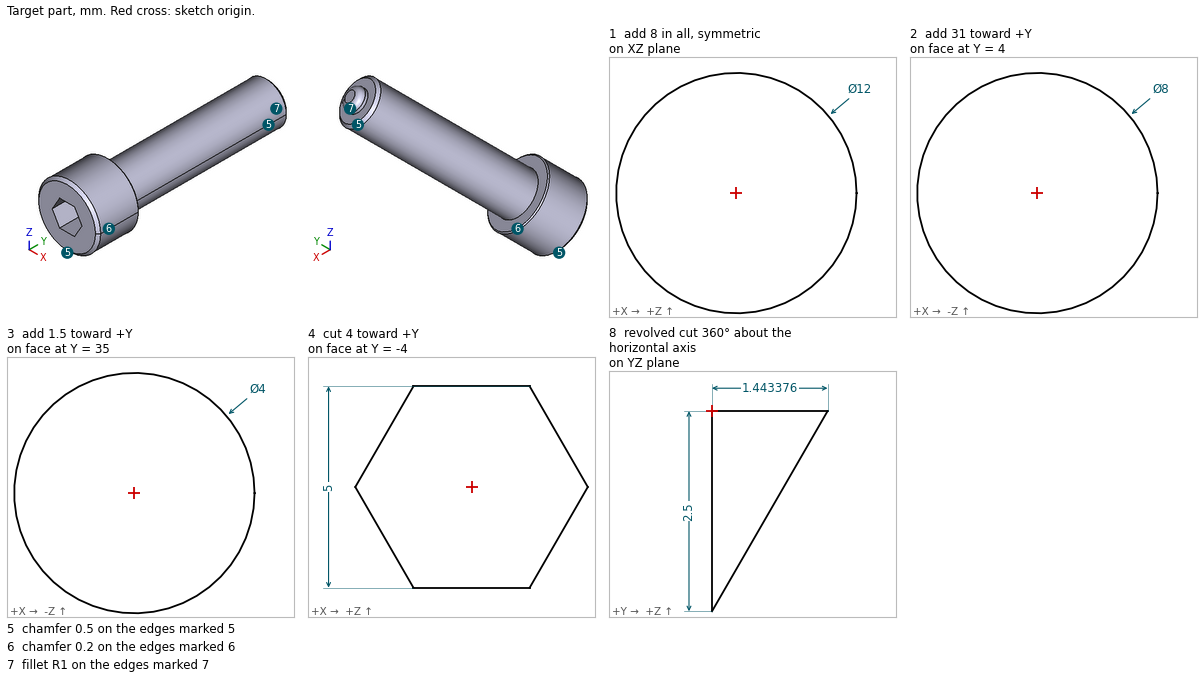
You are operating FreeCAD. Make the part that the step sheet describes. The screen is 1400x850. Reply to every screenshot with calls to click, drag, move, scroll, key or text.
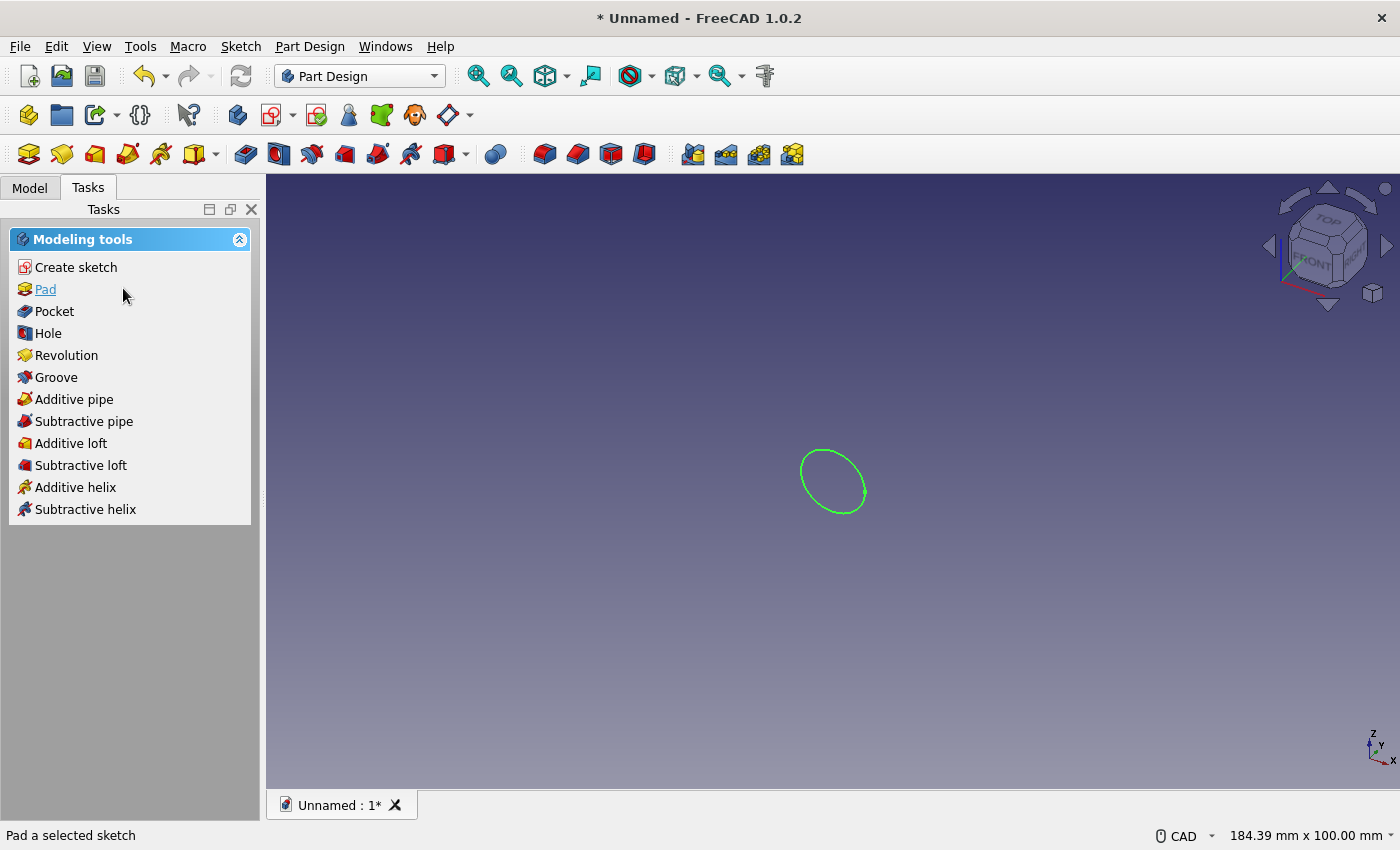
click(29, 154)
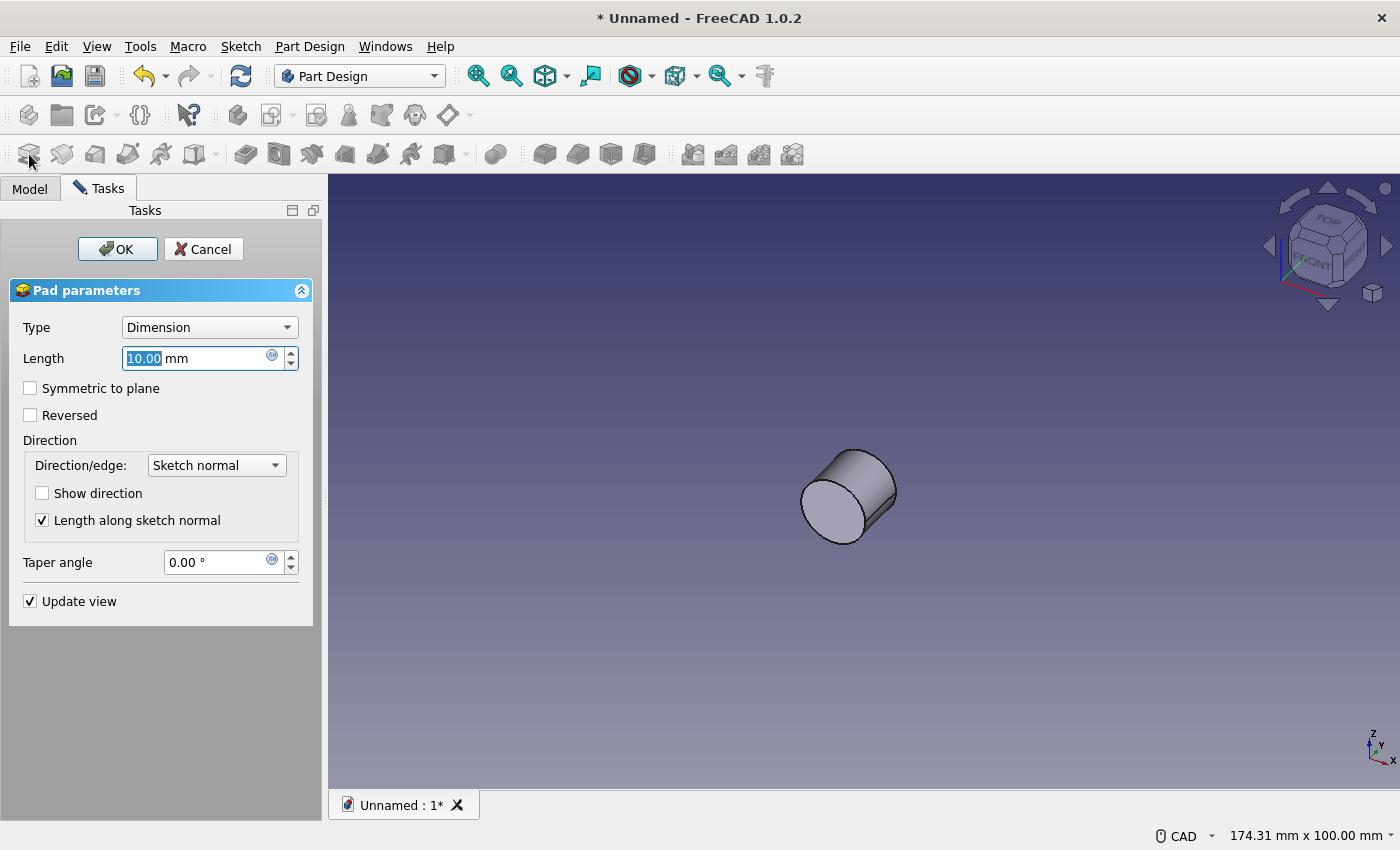
text(8)
key(Tab)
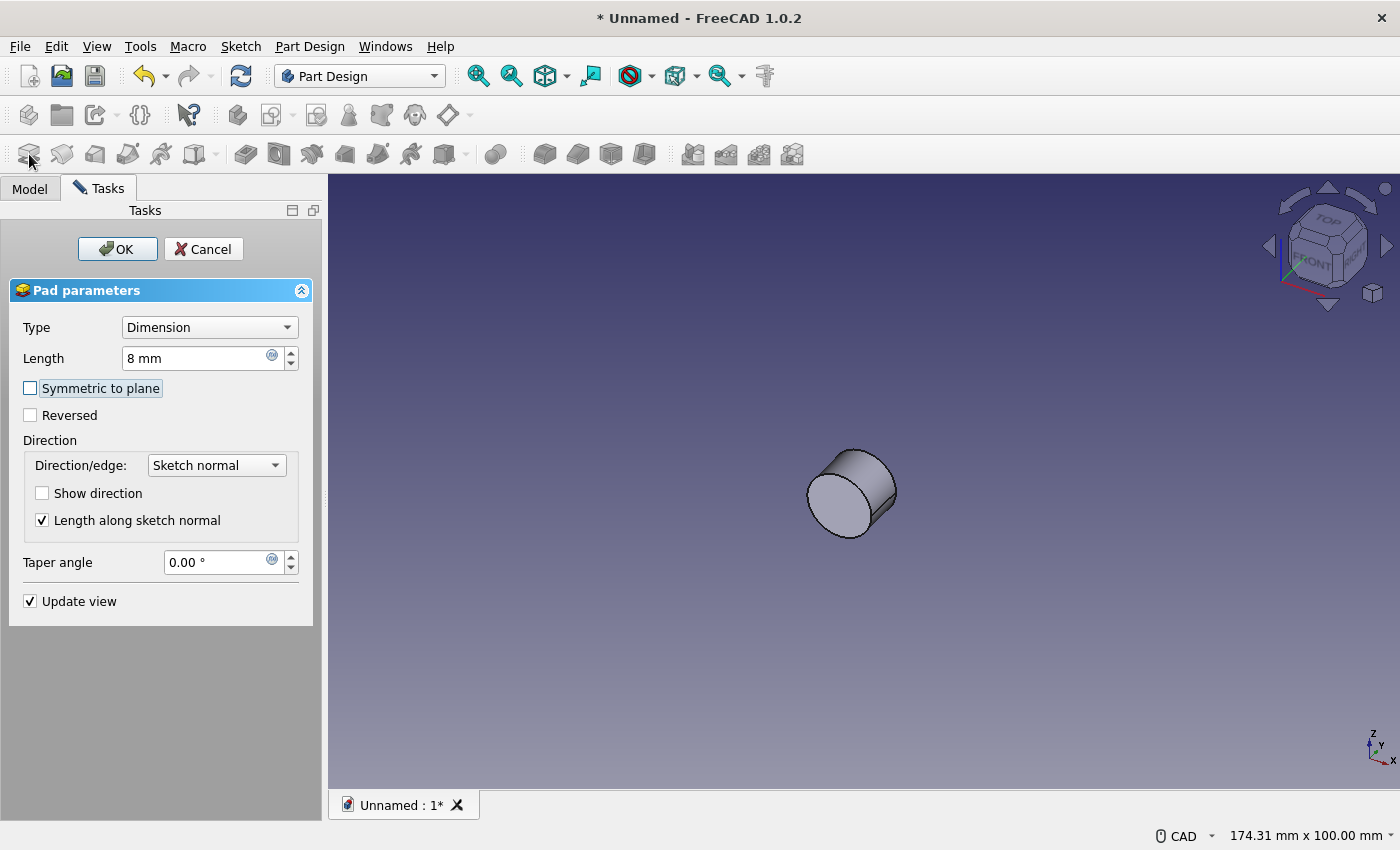
click(31, 388)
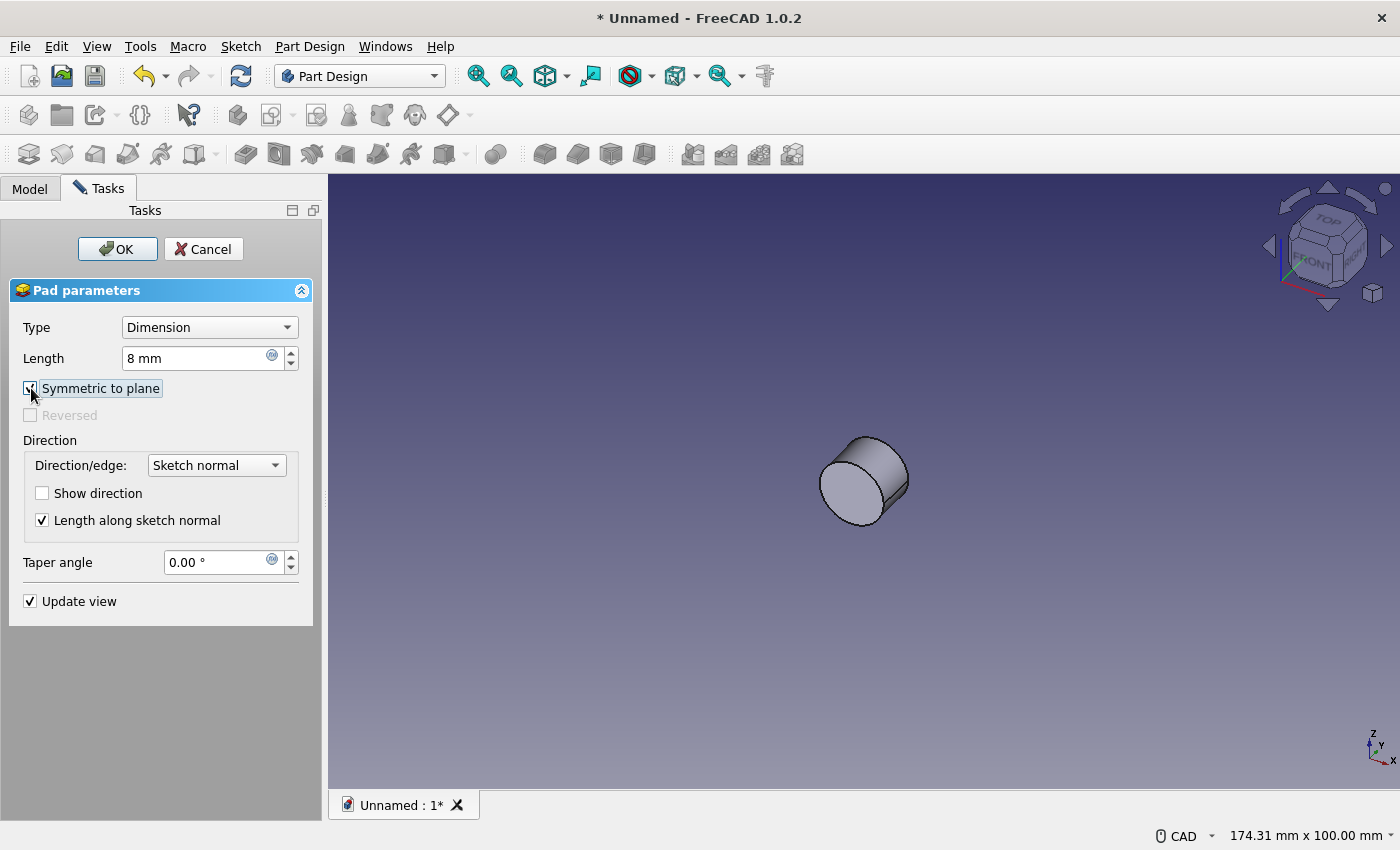
click(118, 249)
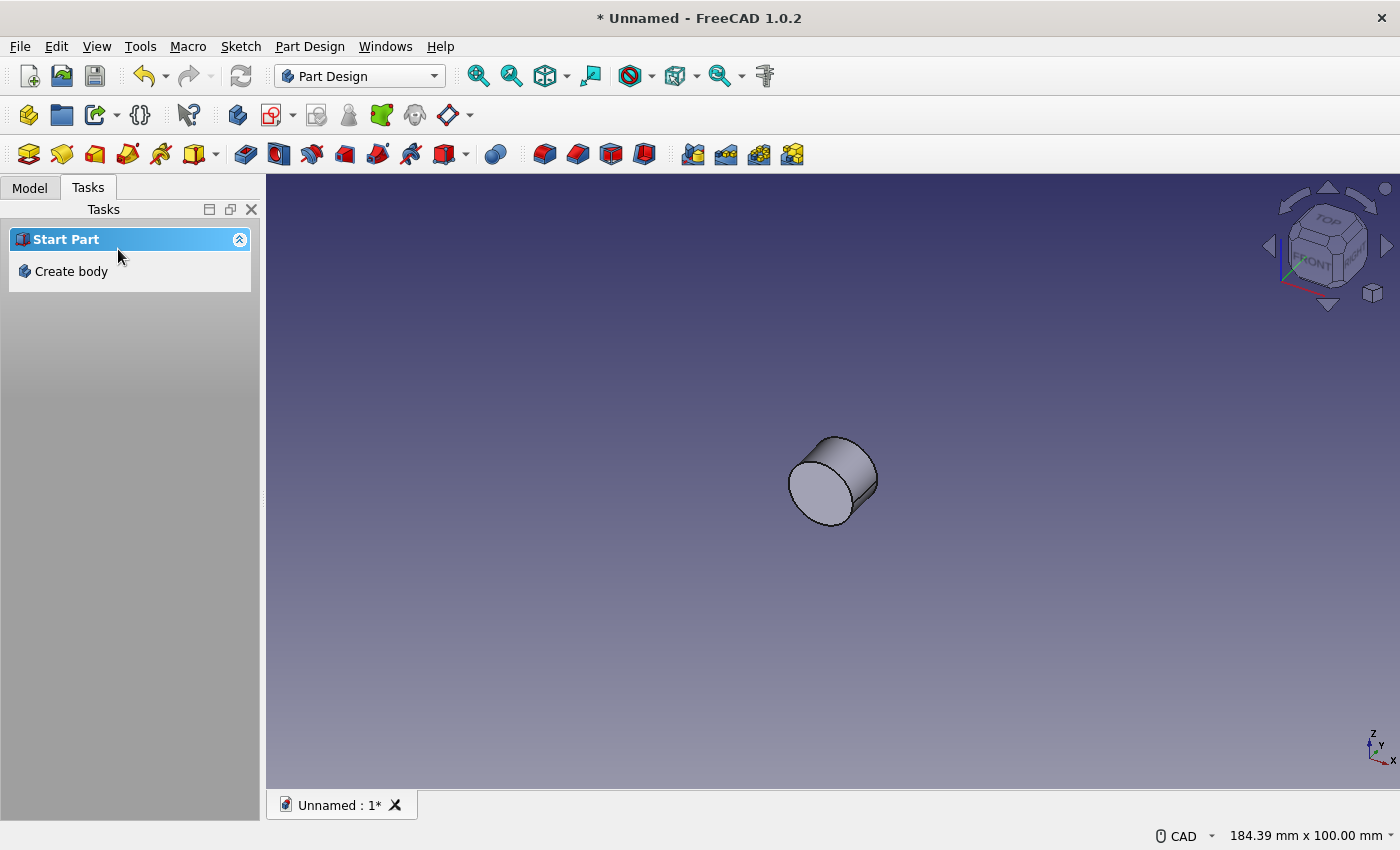
key(v)
key(f)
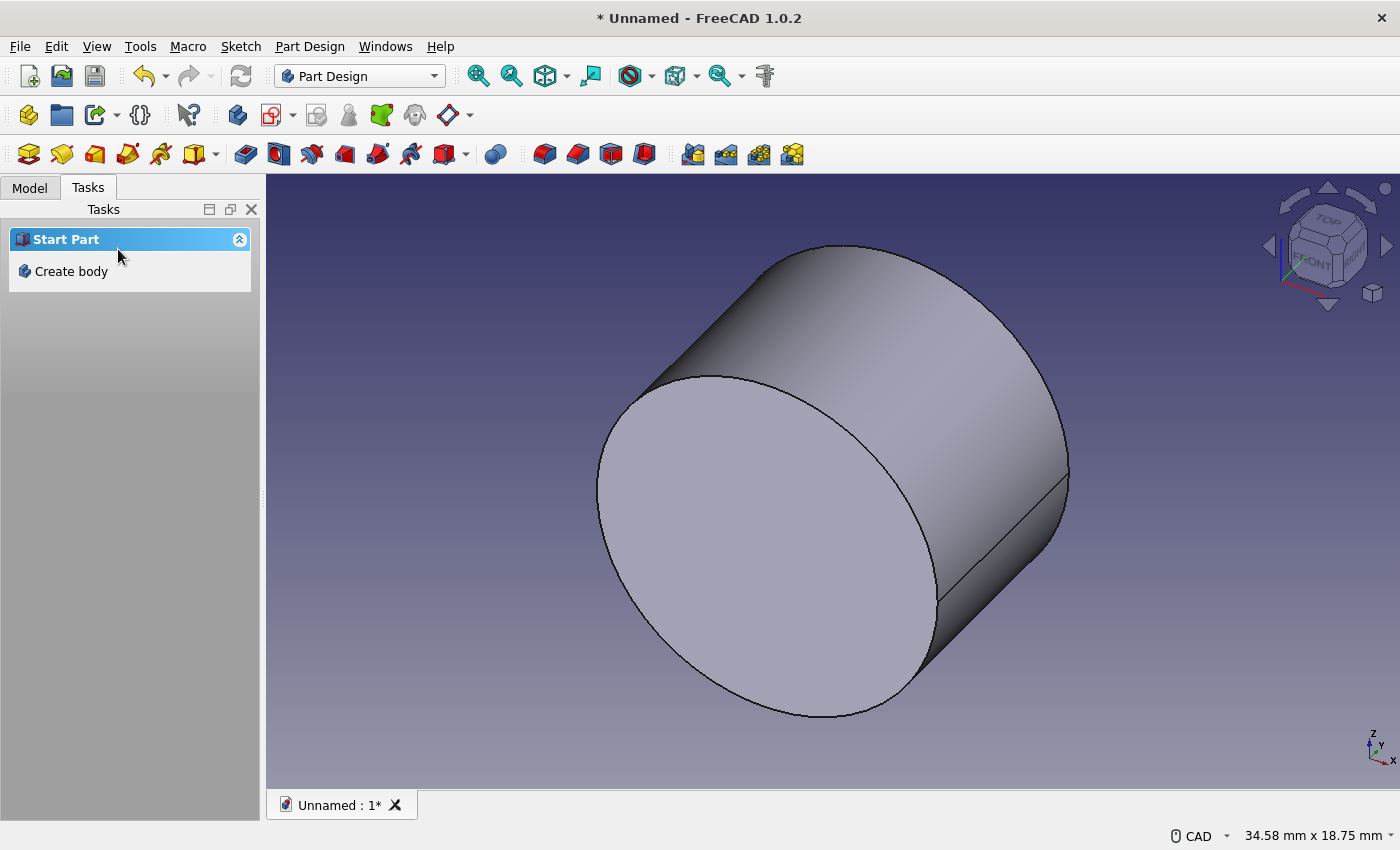
key(4)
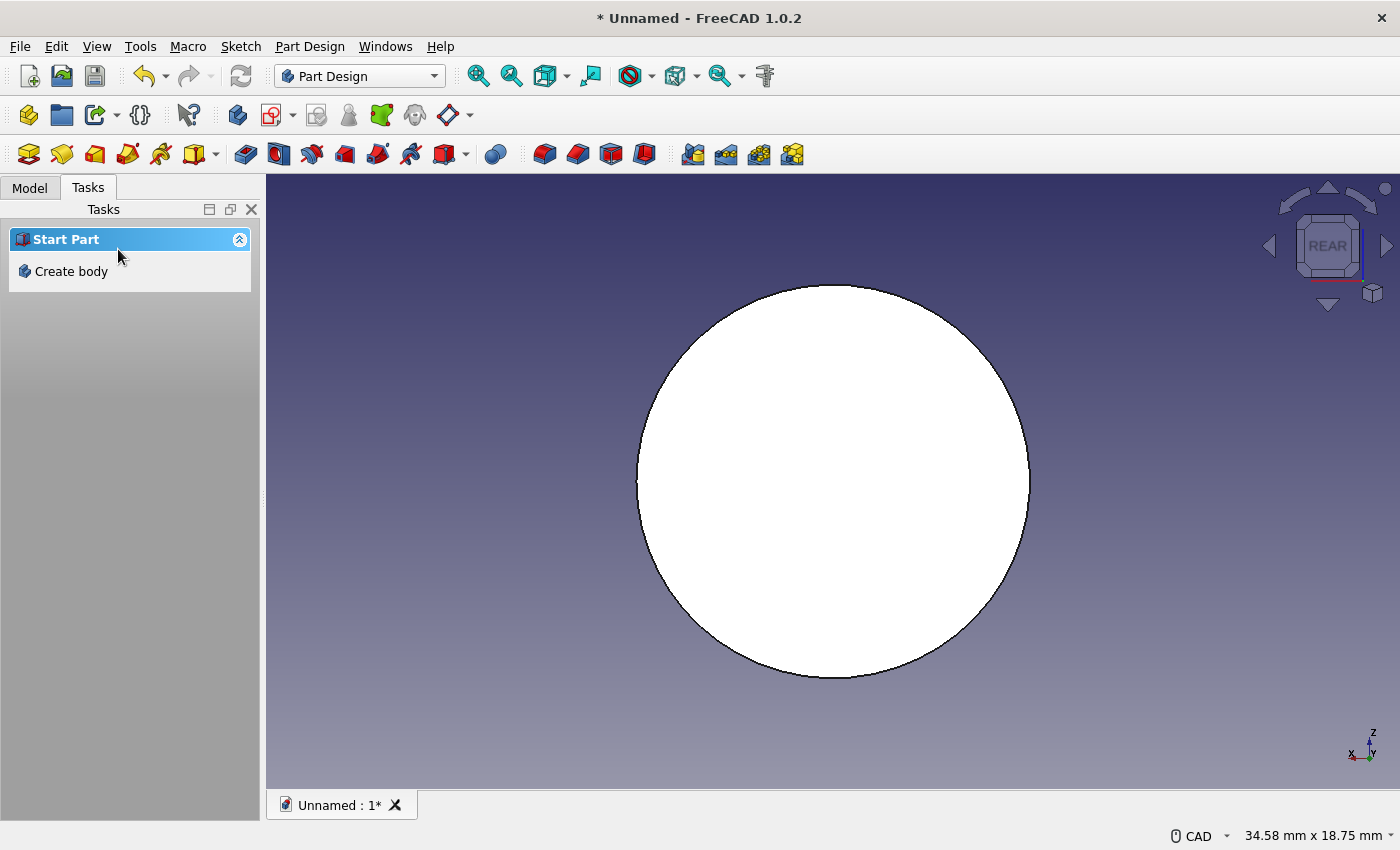
click(833, 481)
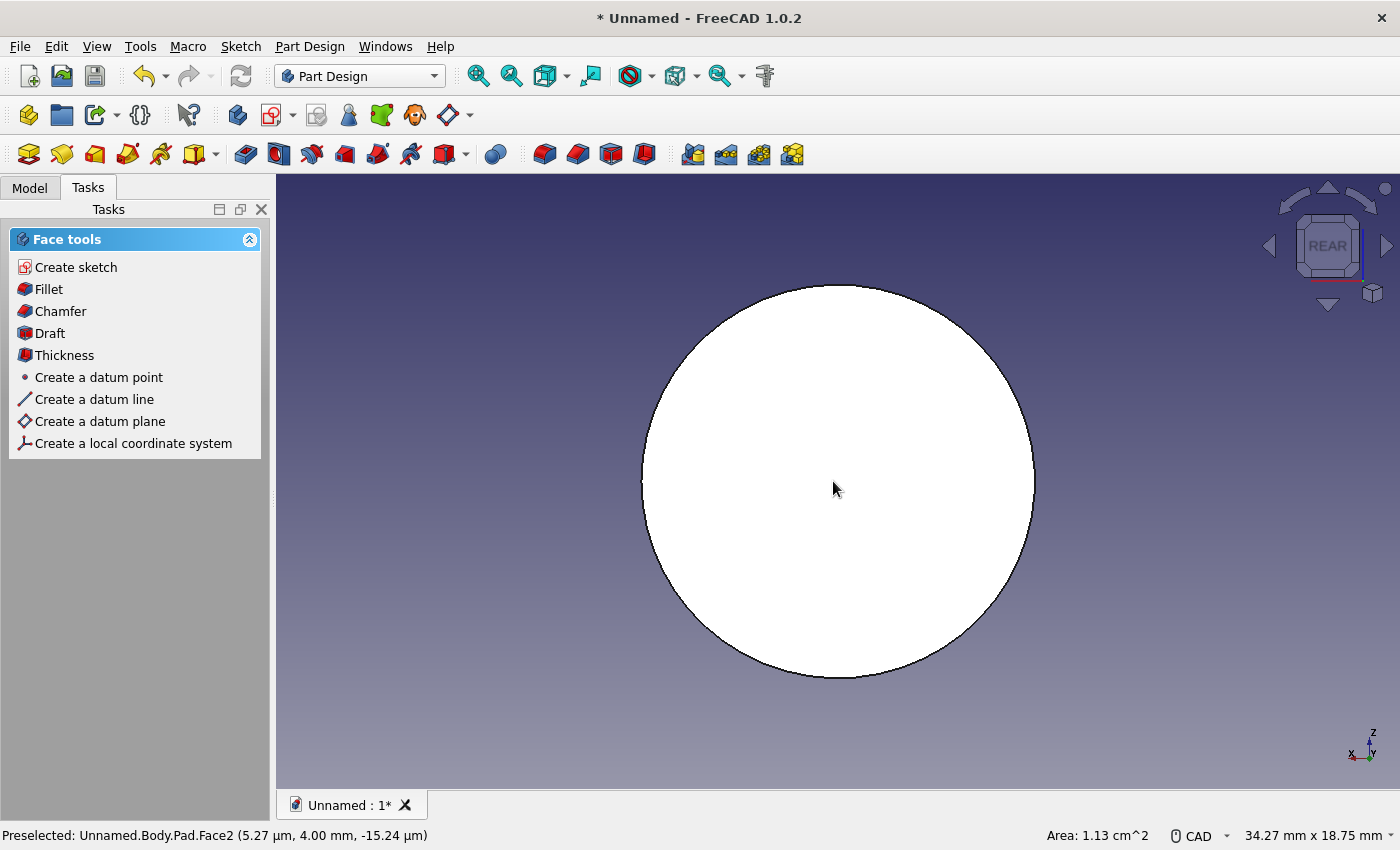
click(270, 116)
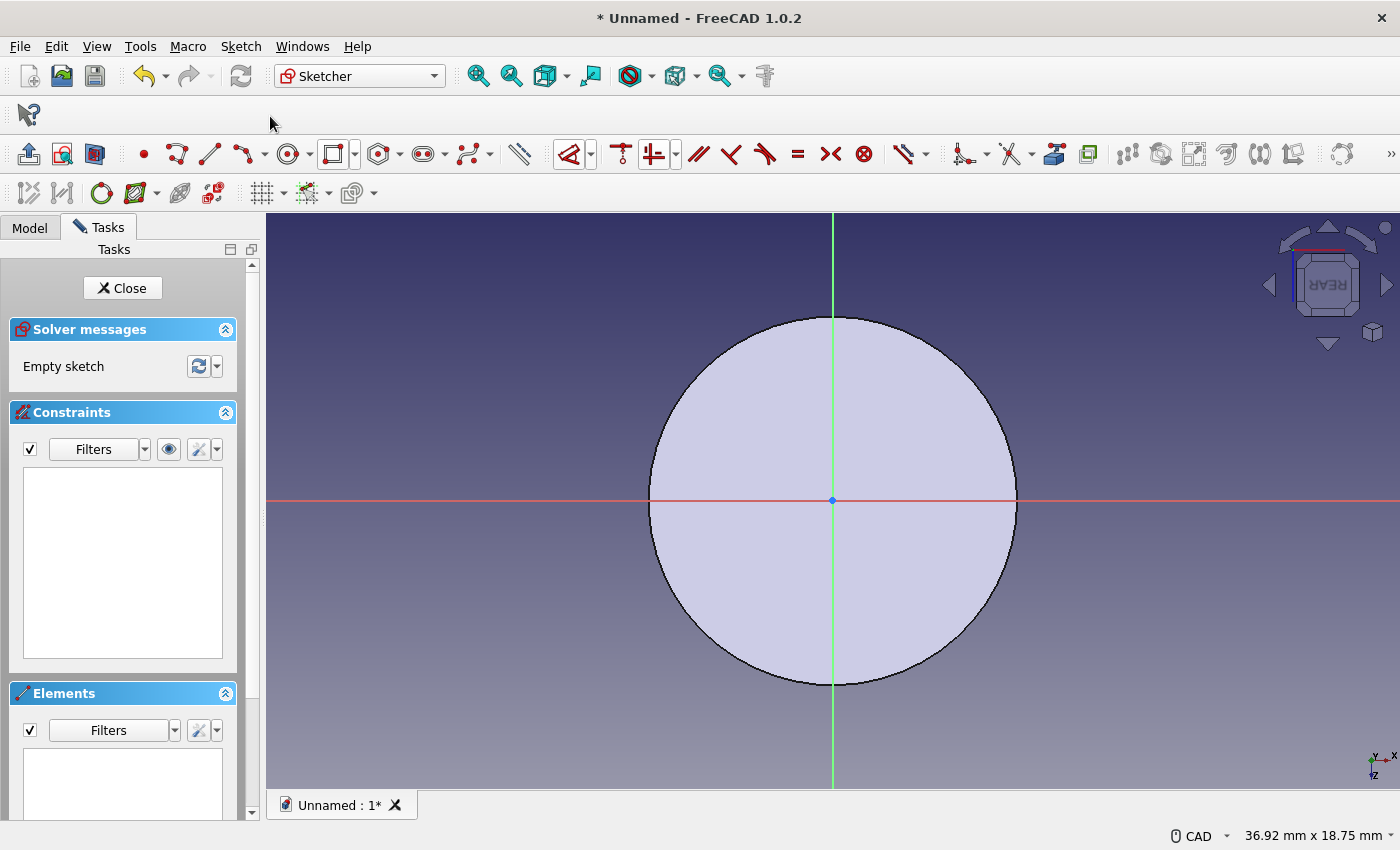
scroll(972, 501, up, 2)